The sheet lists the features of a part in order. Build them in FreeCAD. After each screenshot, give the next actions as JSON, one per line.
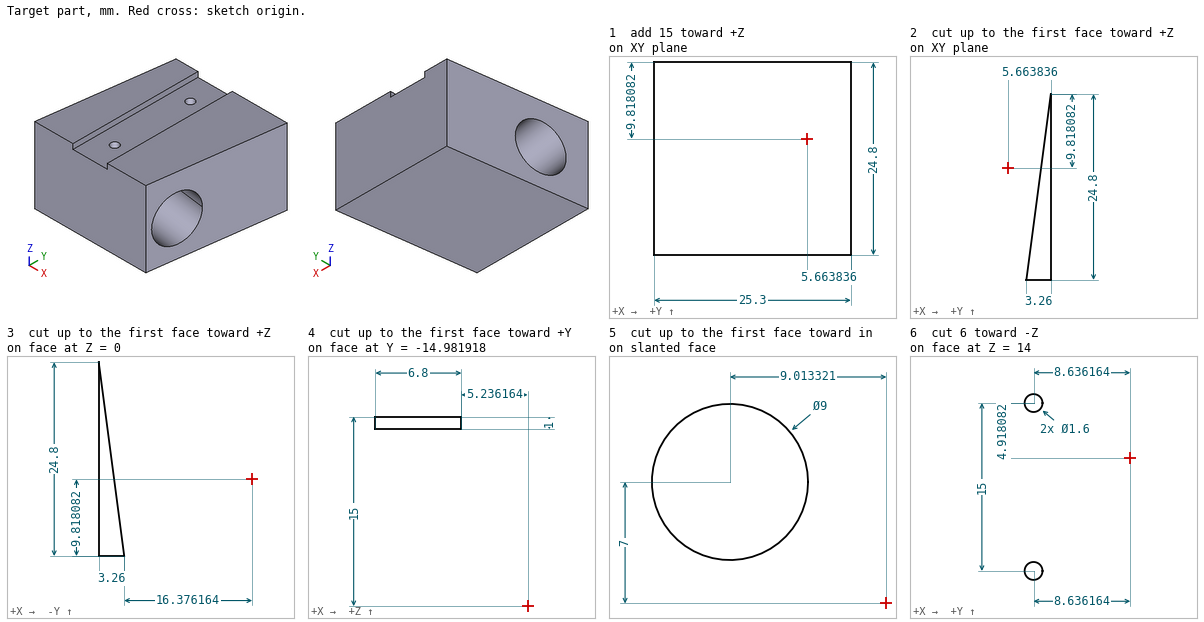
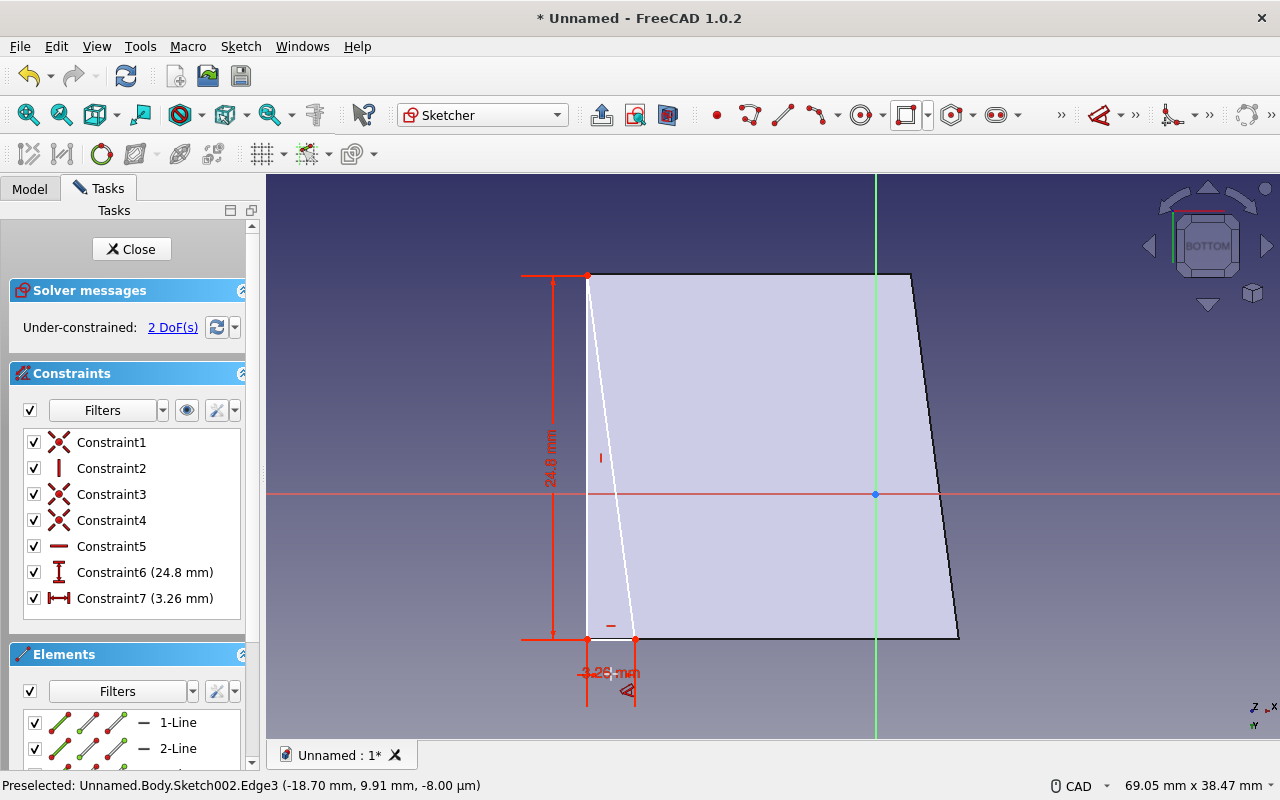
{"action": "left_click", "coordinate": [635, 640]}
{"action": "left_click", "coordinate": [910, 567]}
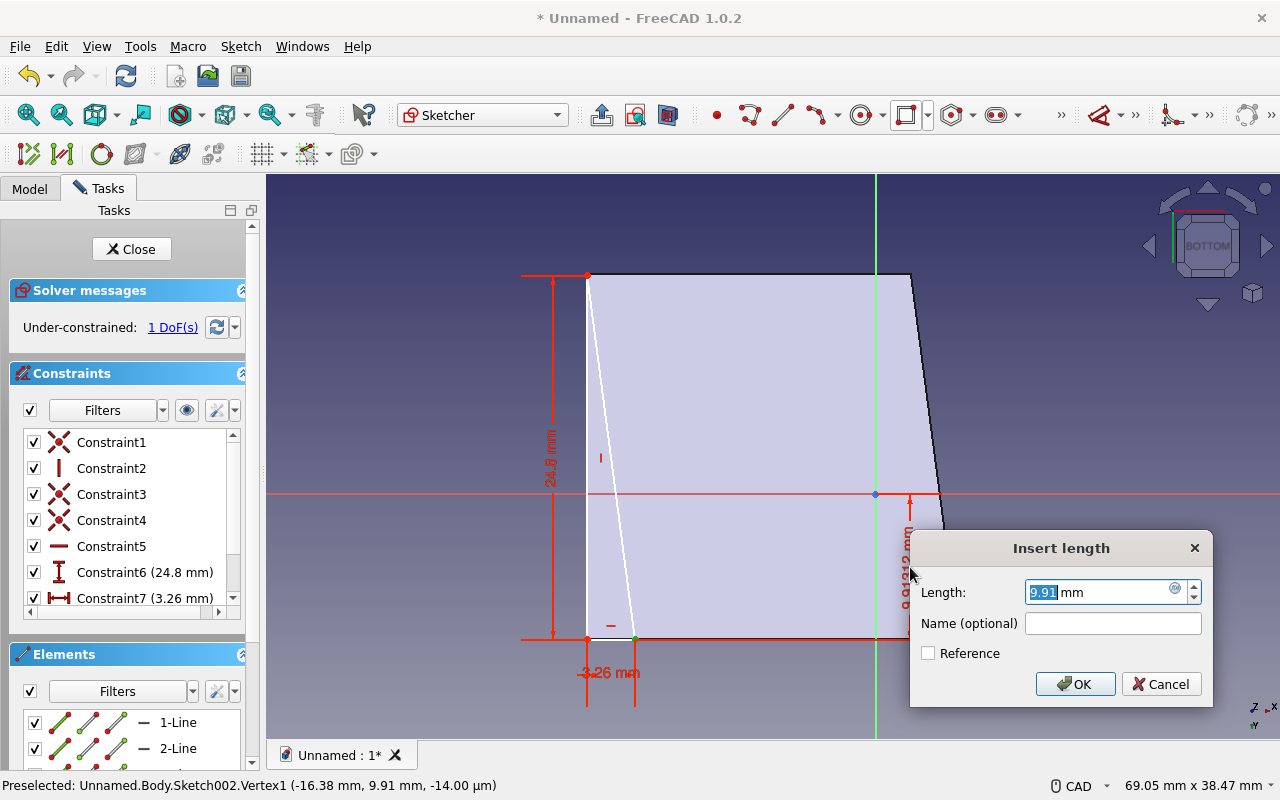
{"action": "type", "text": "9.818082"}
{"action": "key", "text": "Return"}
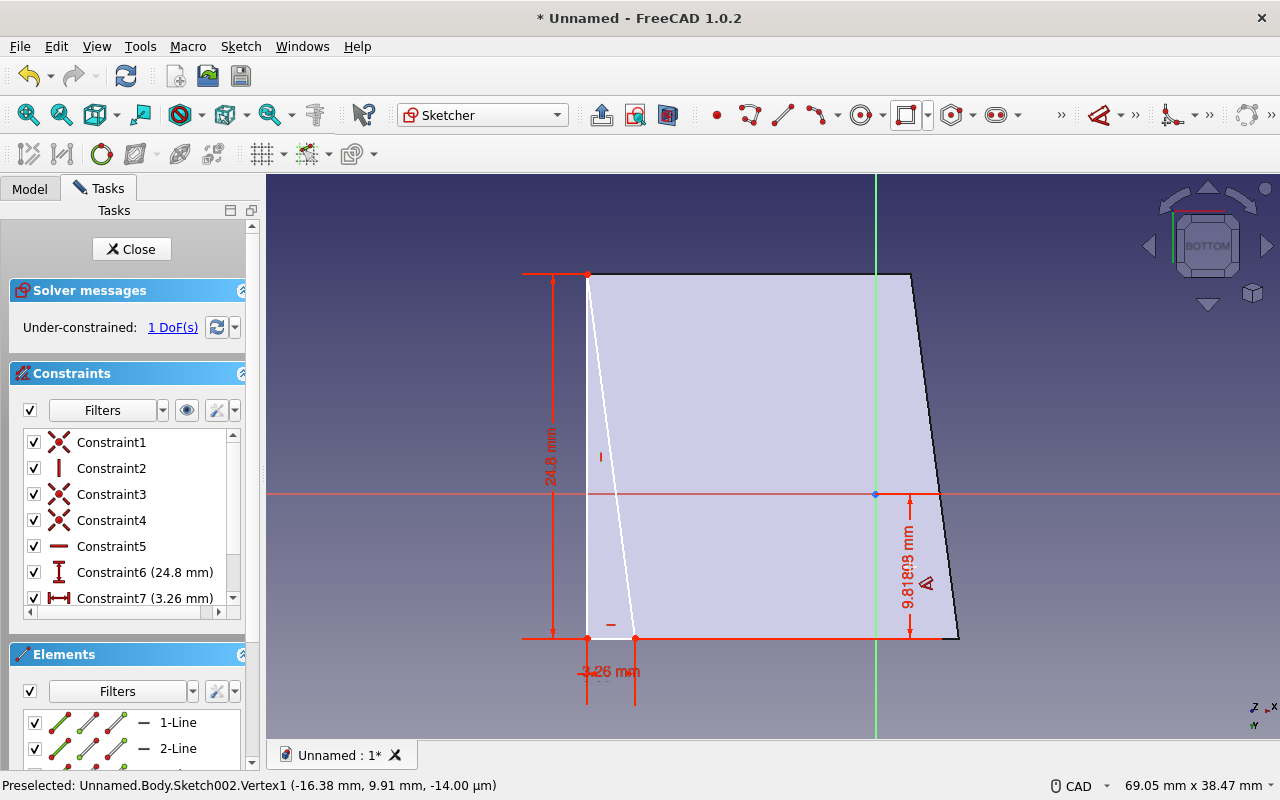
{"action": "left_click", "coordinate": [635, 639]}
{"action": "left_click", "coordinate": [755, 673]}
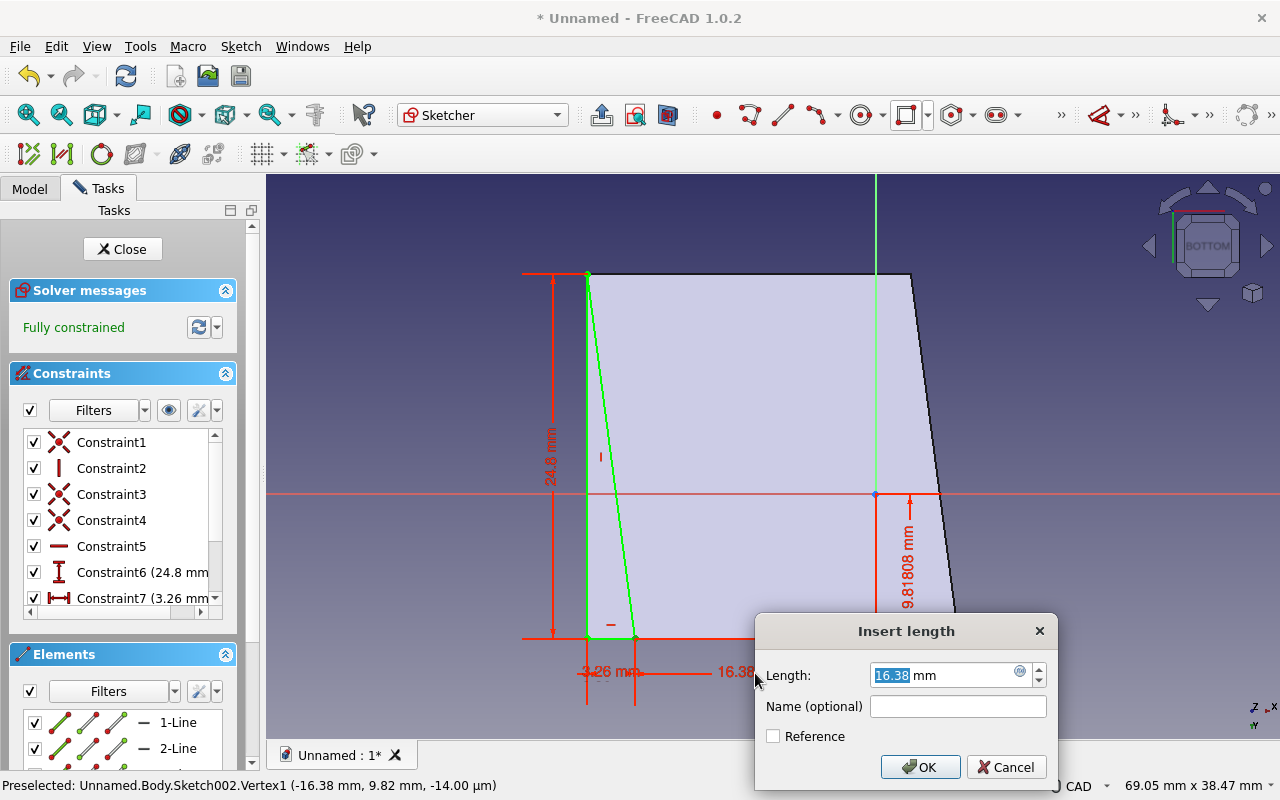
{"action": "type", "text": "16.376164"}
{"action": "key", "text": "Return"}
{"action": "key", "text": "Escape"}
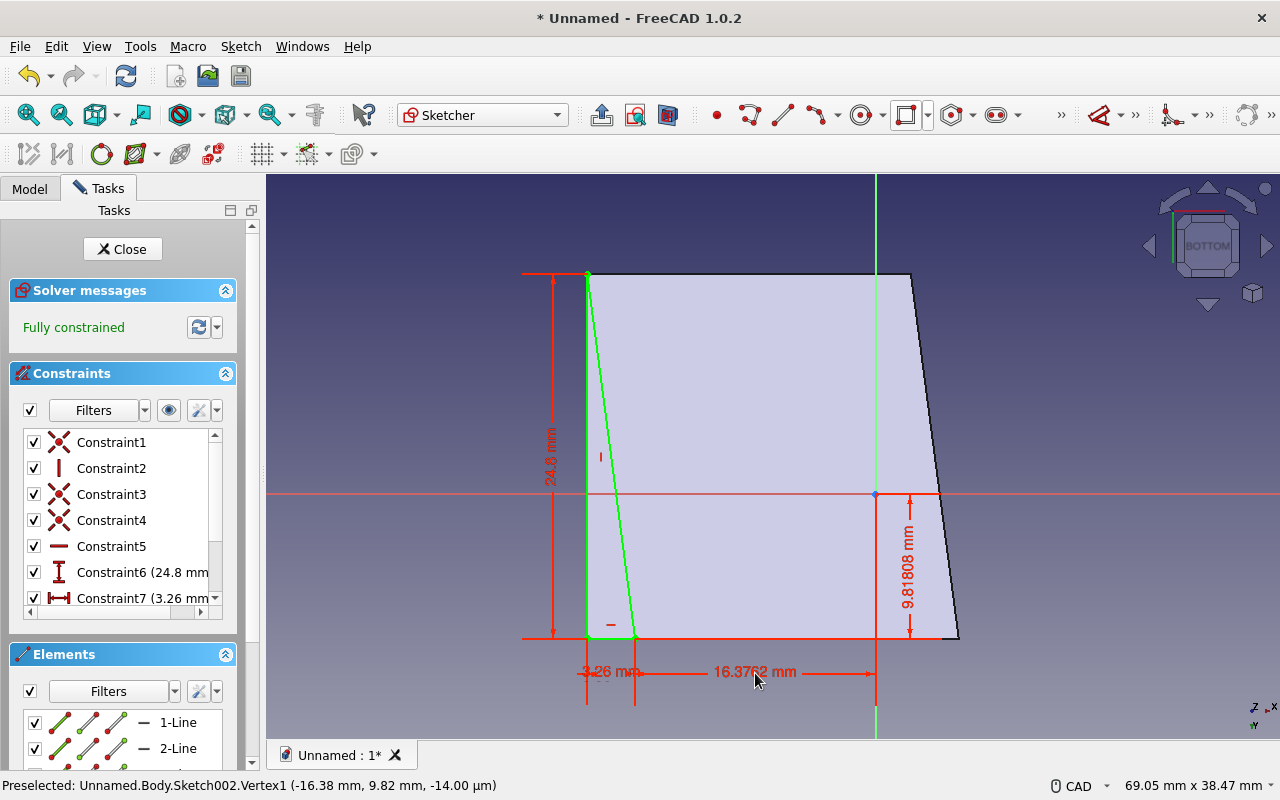
{"action": "left_click", "coordinate": [123, 249]}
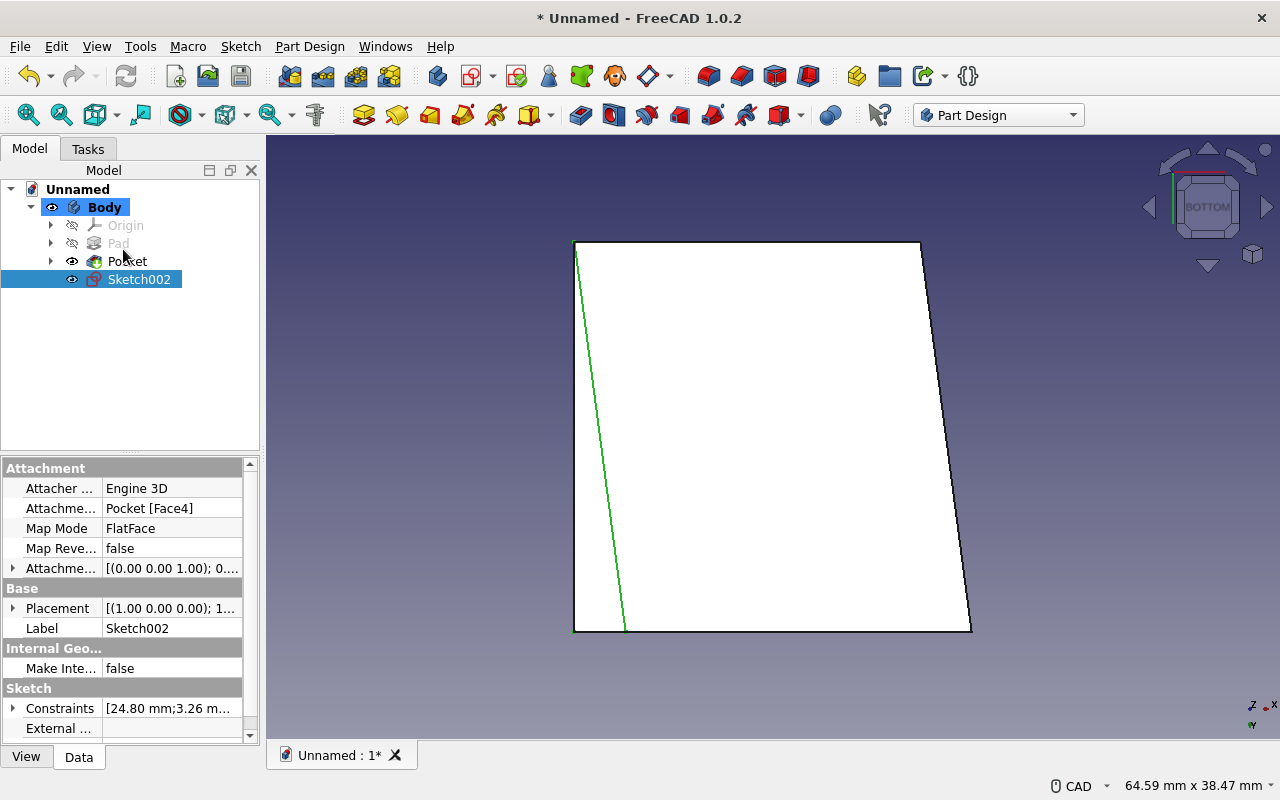
{"action": "left_click", "coordinate": [581, 116]}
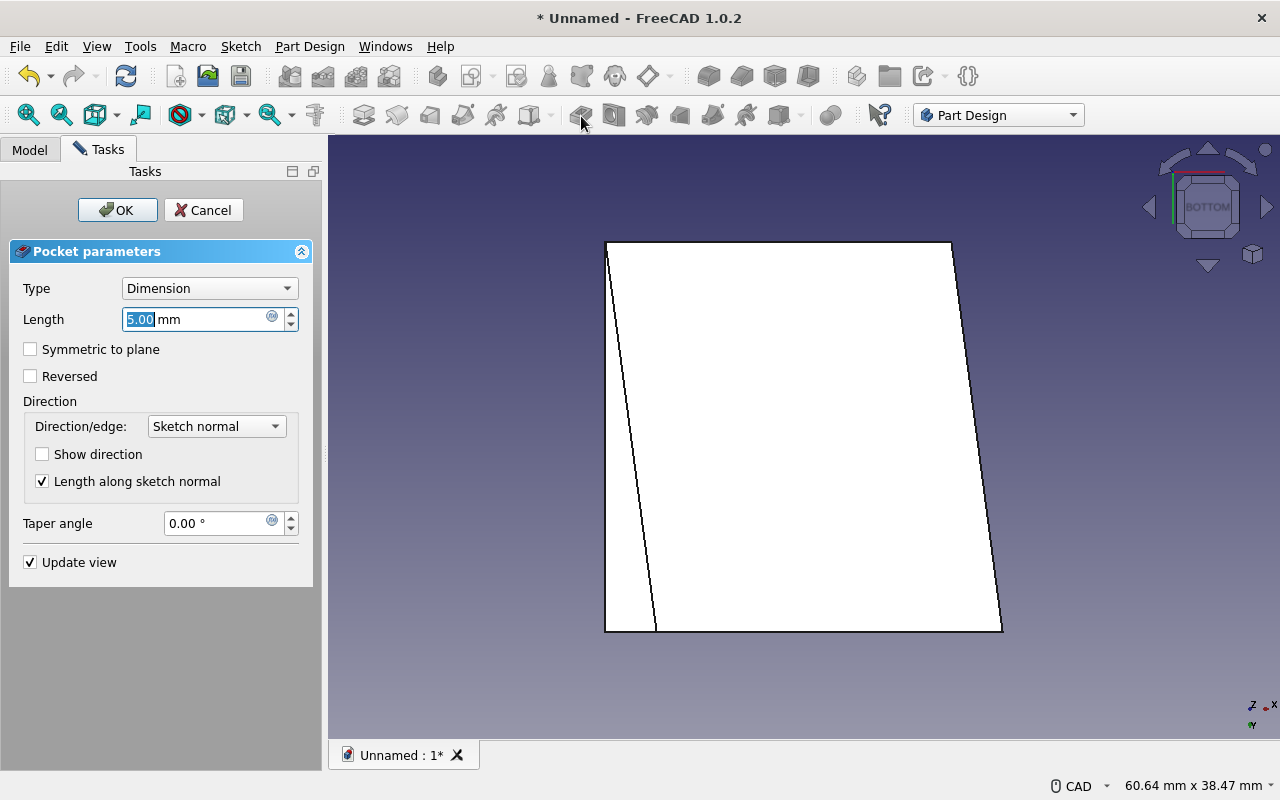
{"action": "left_click", "coordinate": [210, 288]}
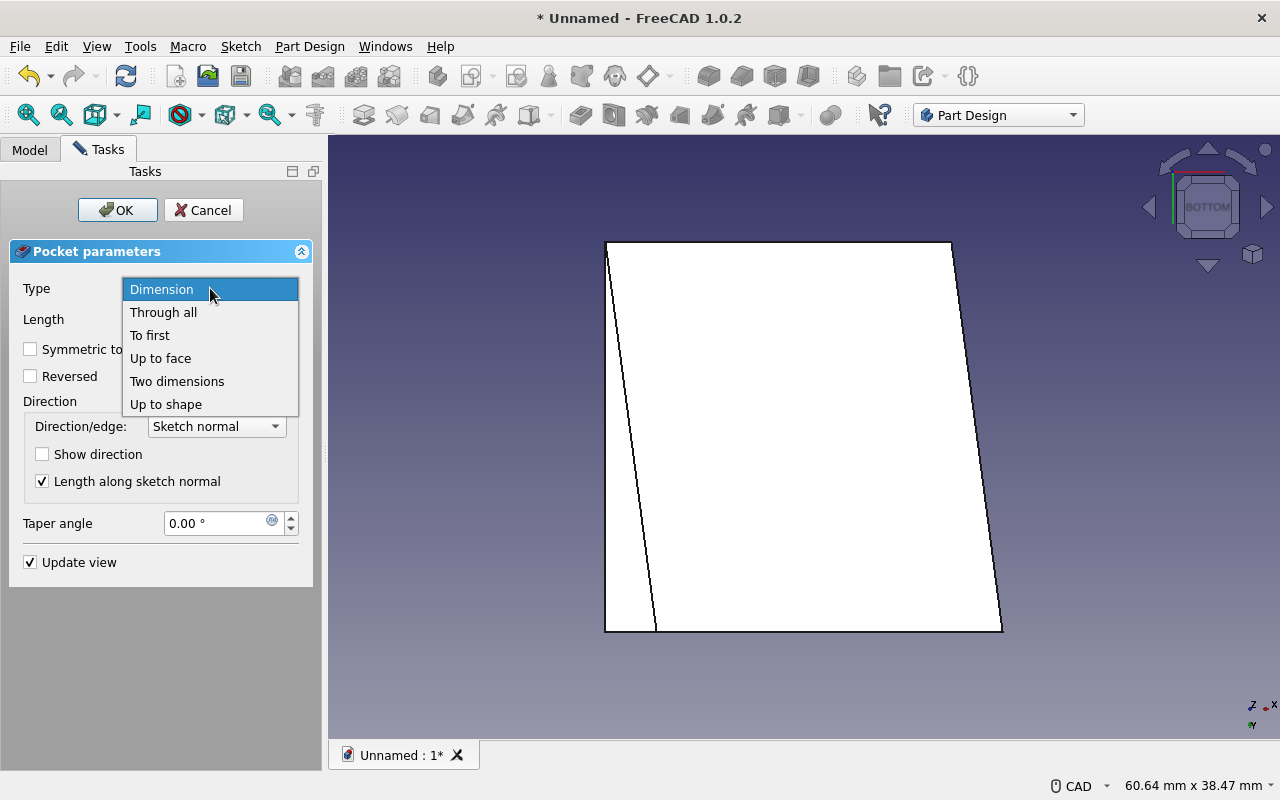
{"action": "left_click", "coordinate": [208, 336]}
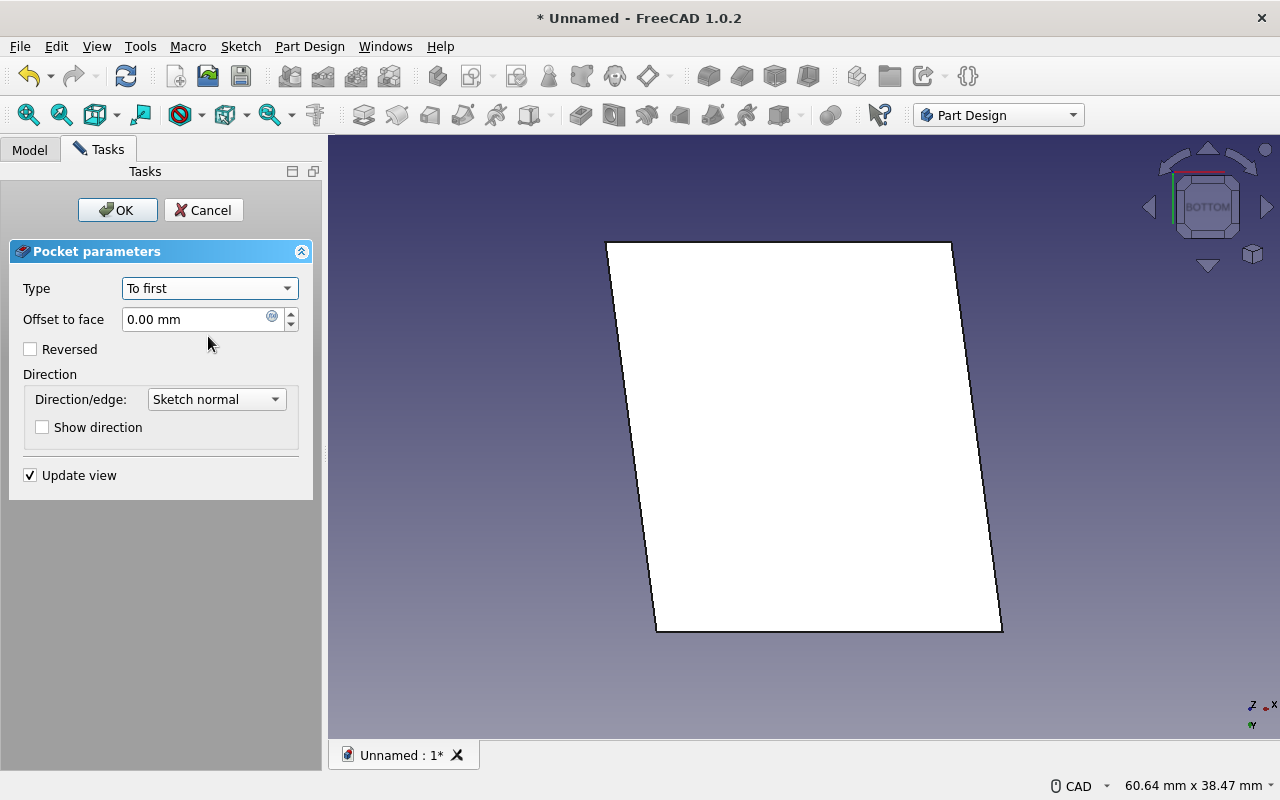
{"action": "left_click", "coordinate": [118, 210]}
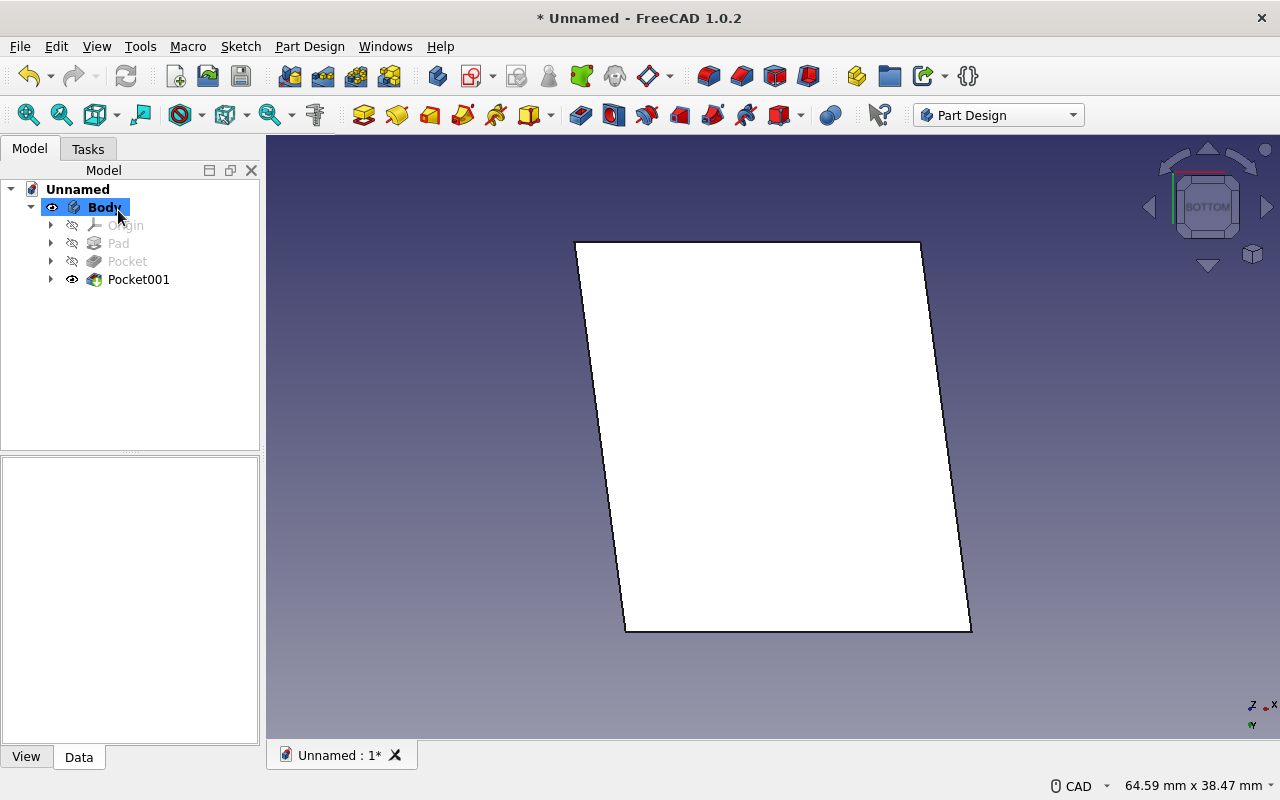
{"action": "key", "text": "0"}